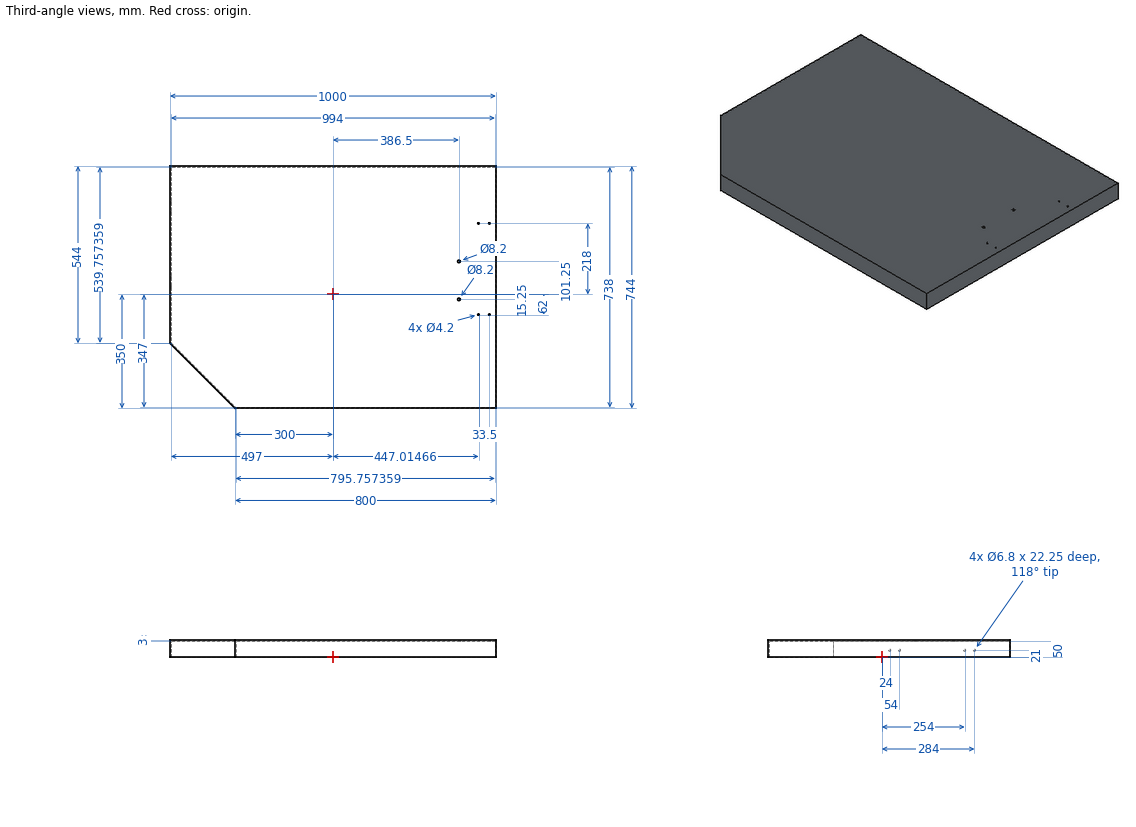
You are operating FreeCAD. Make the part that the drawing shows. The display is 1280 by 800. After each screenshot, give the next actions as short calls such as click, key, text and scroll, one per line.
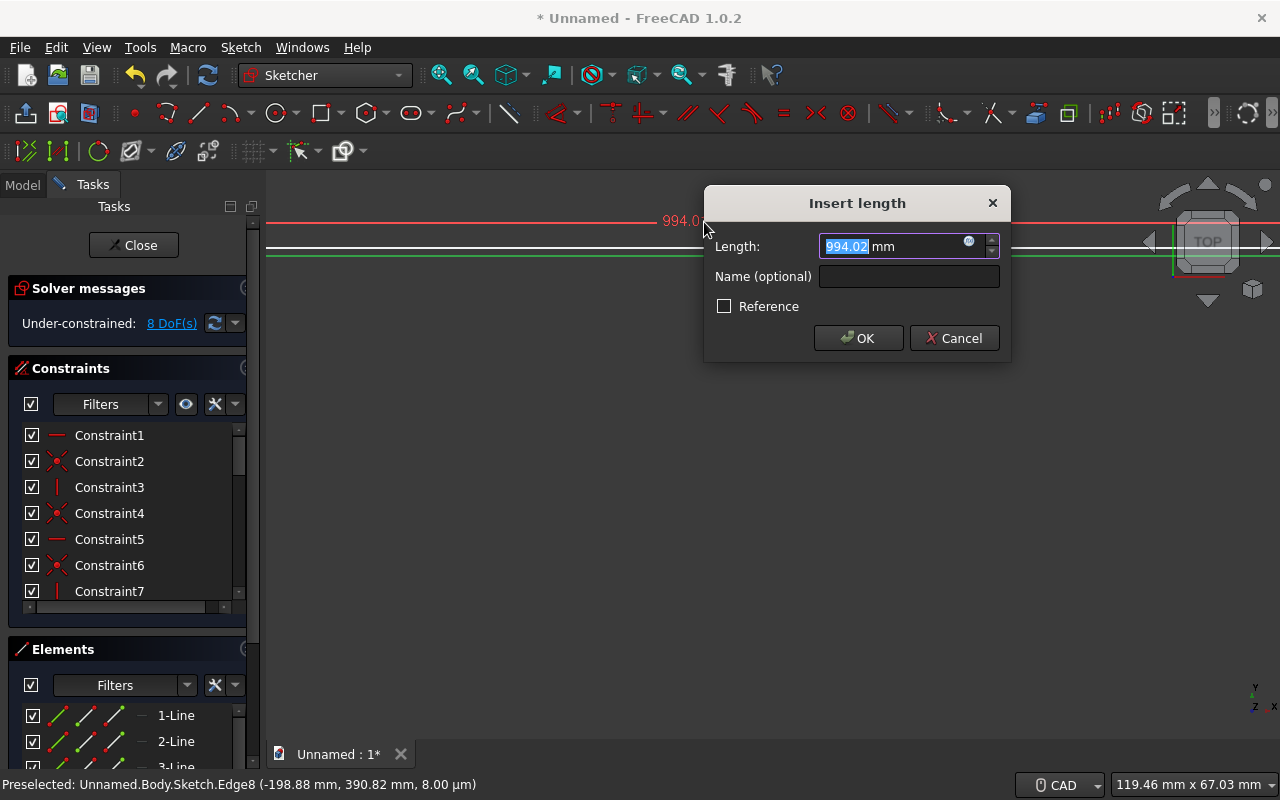
text(994)
key(Return)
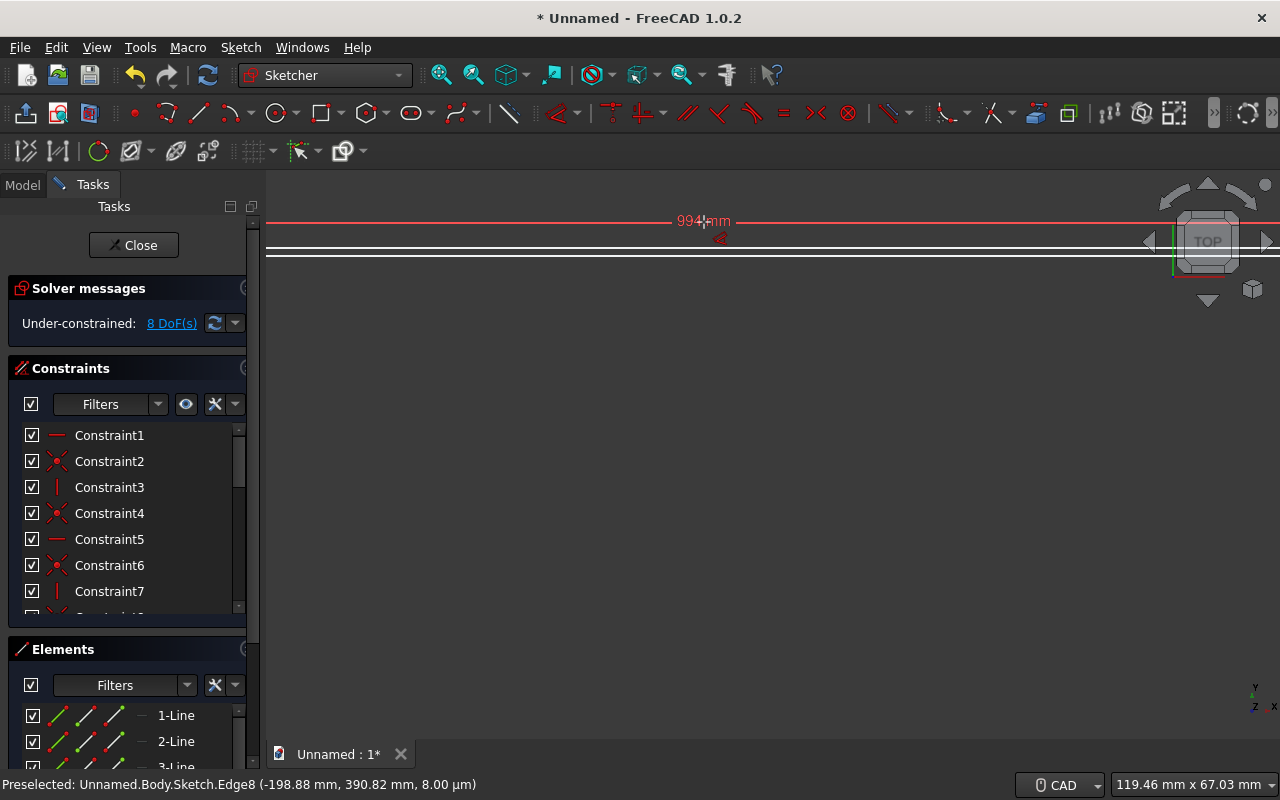
scroll(603, 265, down, 14)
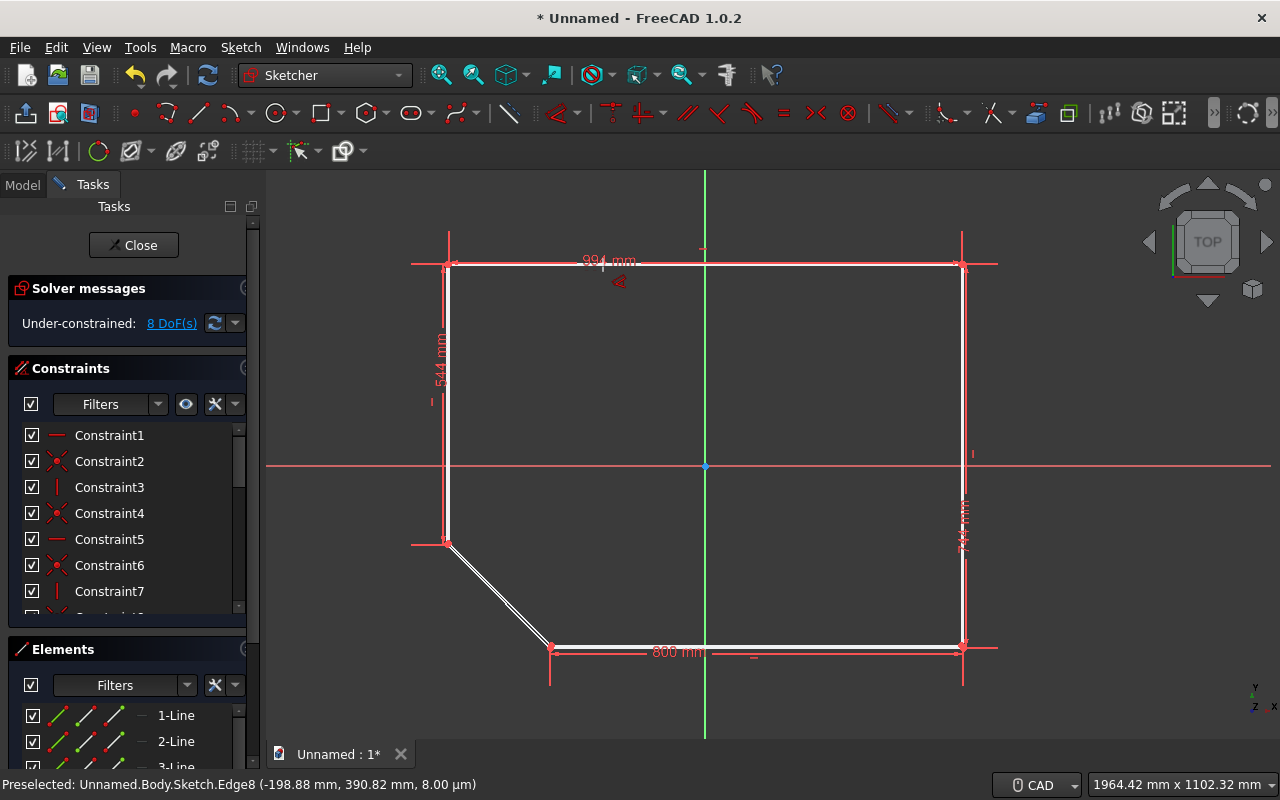
scroll(962, 379, up, 12)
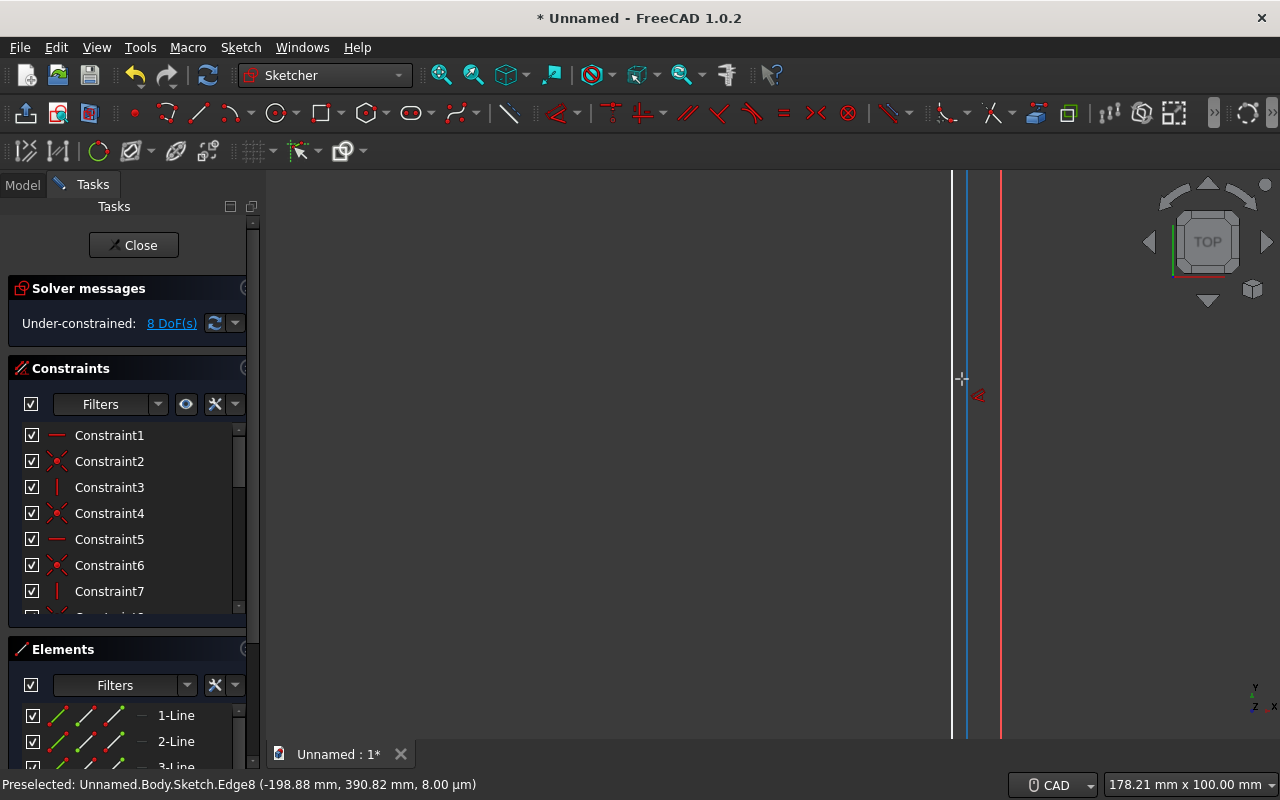
click(952, 374)
click(986, 454)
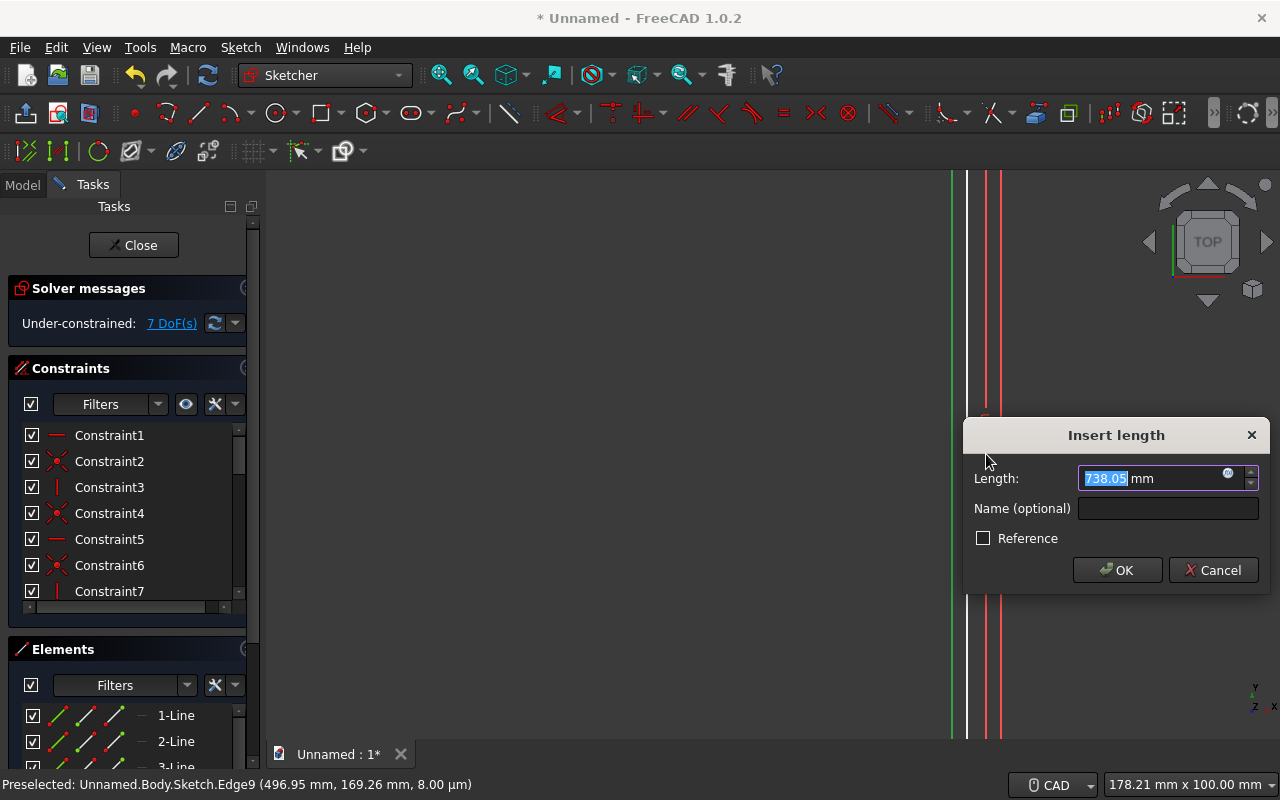
text(738)
key(Return)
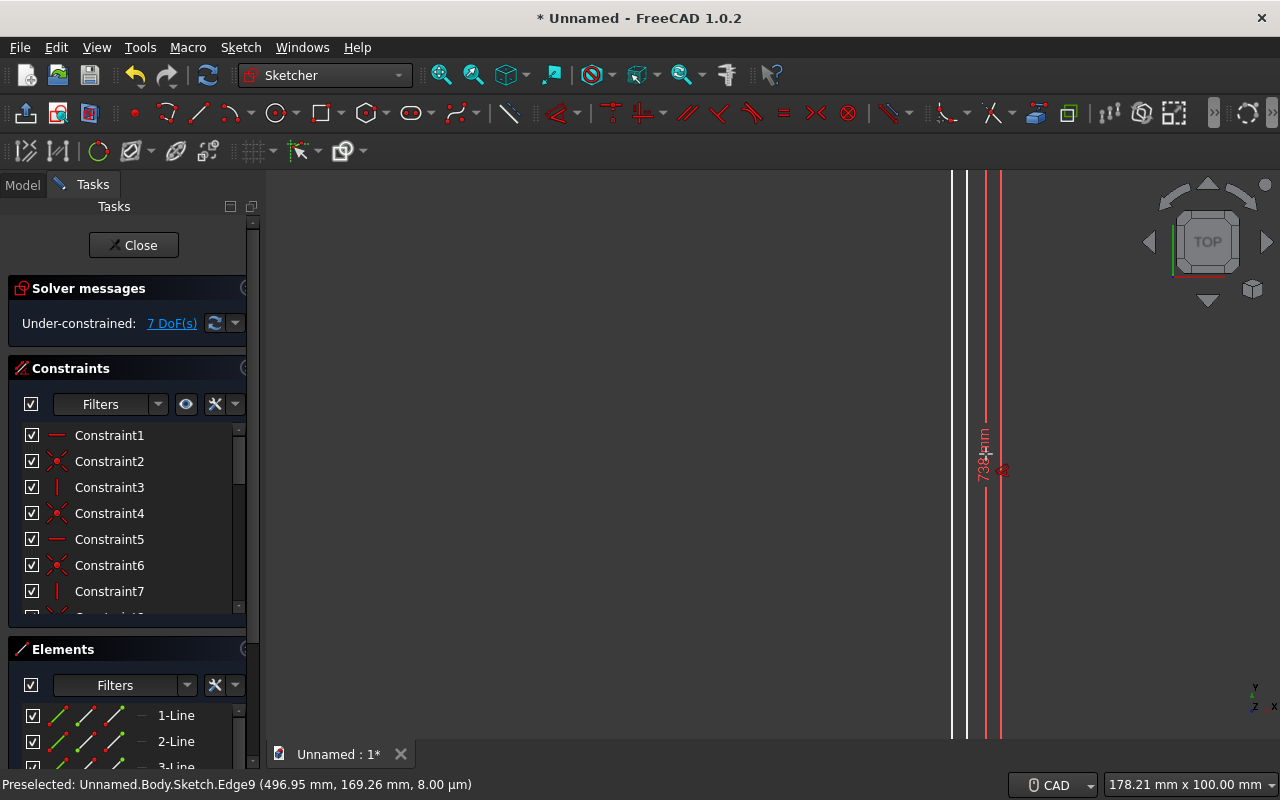
scroll(962, 379, down, 12)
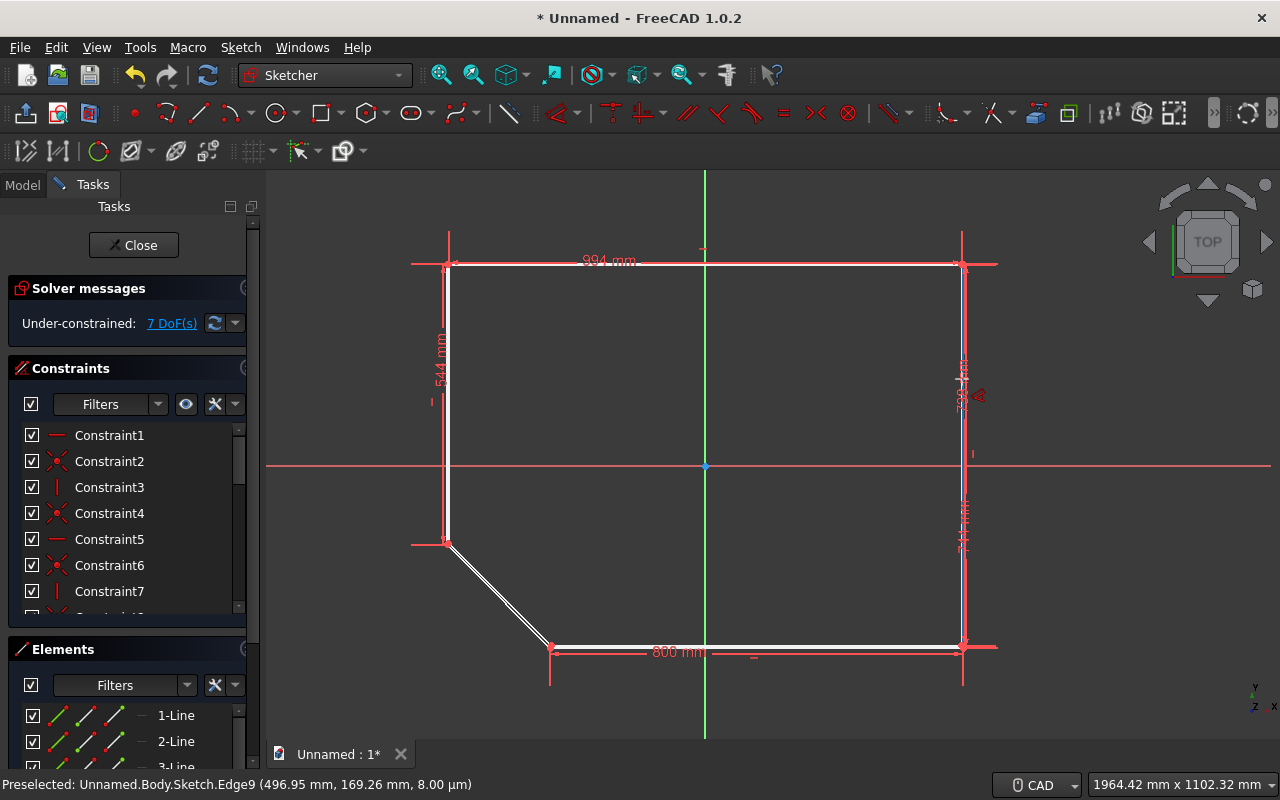
scroll(808, 264, up, 14)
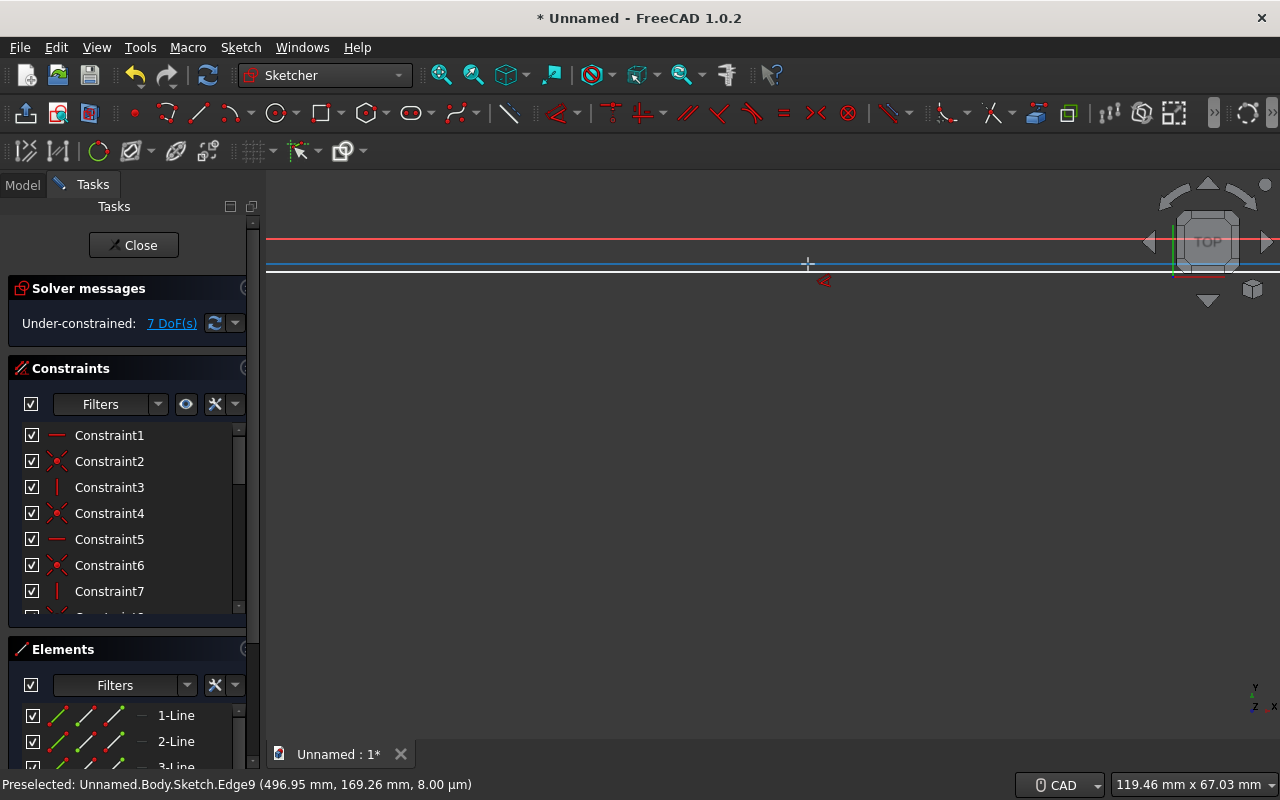
click(804, 264)
click(704, 230)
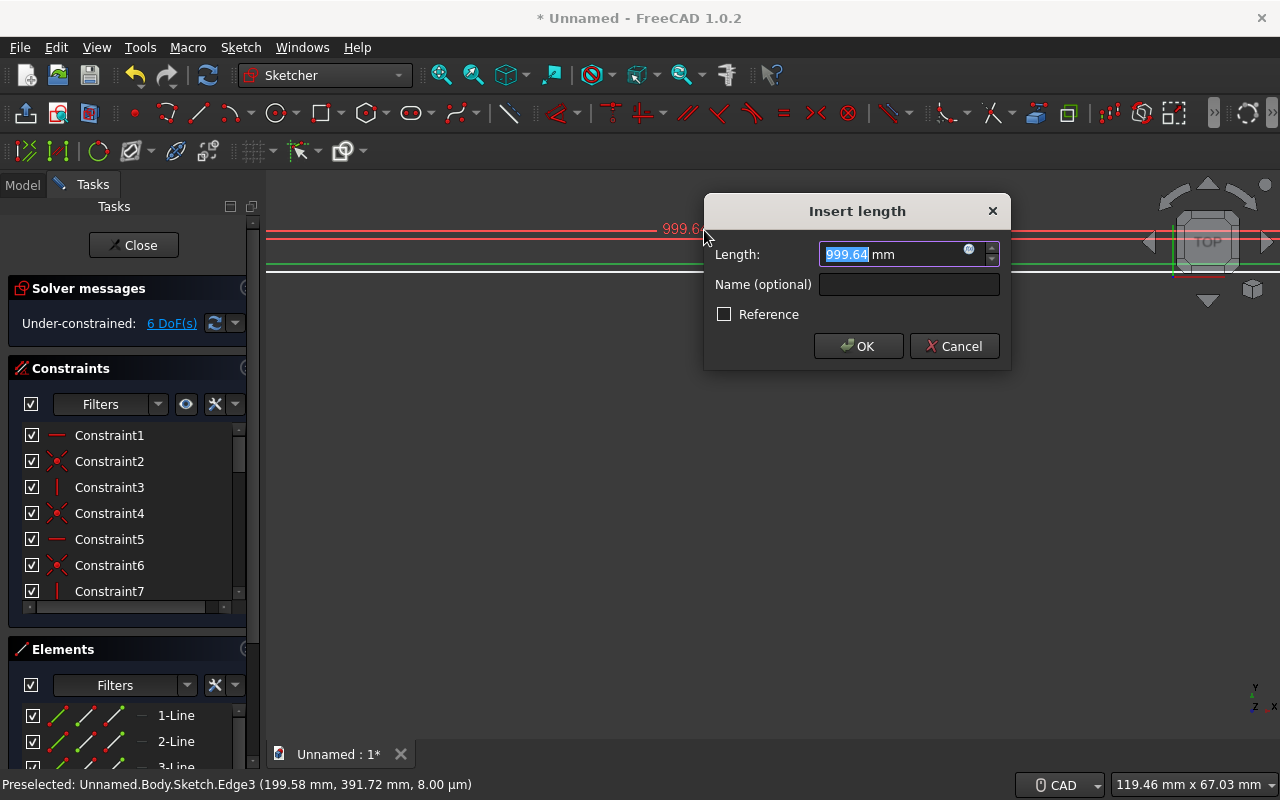
text(1000)
key(Return)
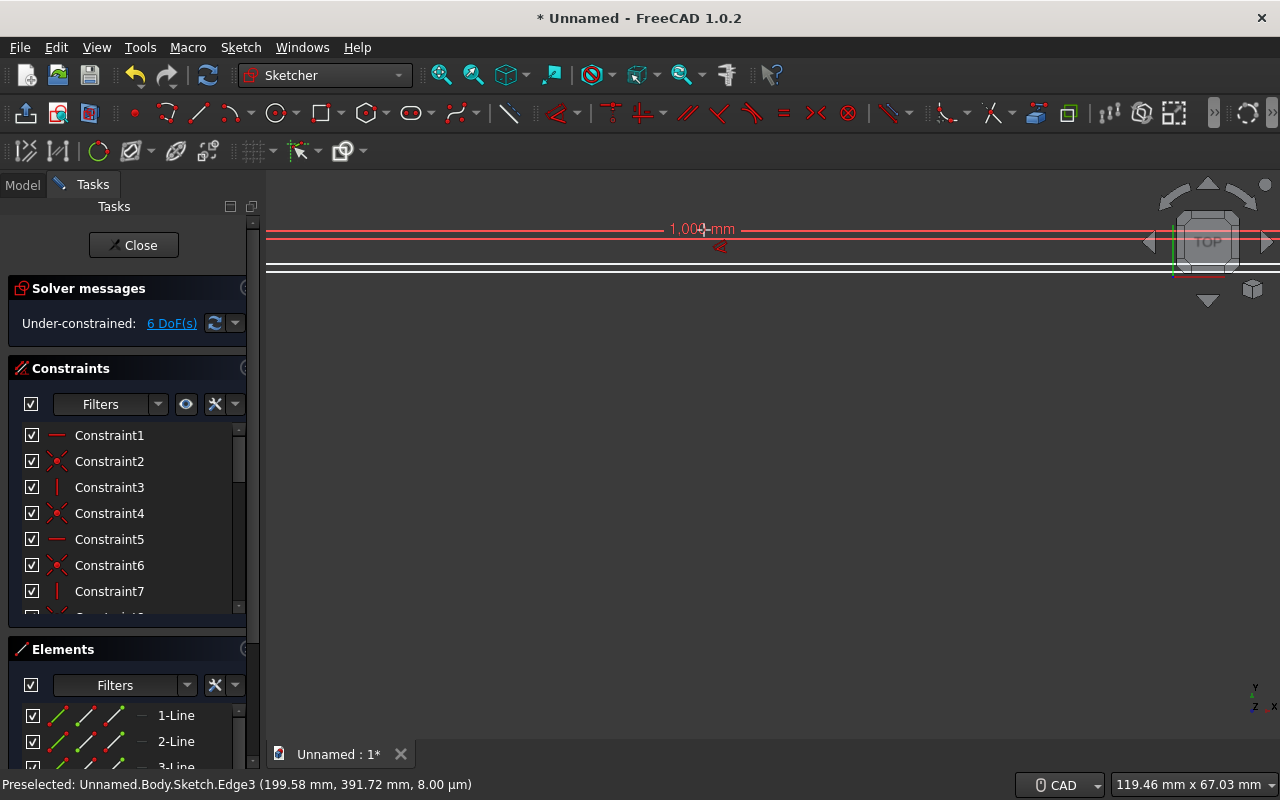
scroll(808, 264, down, 14)